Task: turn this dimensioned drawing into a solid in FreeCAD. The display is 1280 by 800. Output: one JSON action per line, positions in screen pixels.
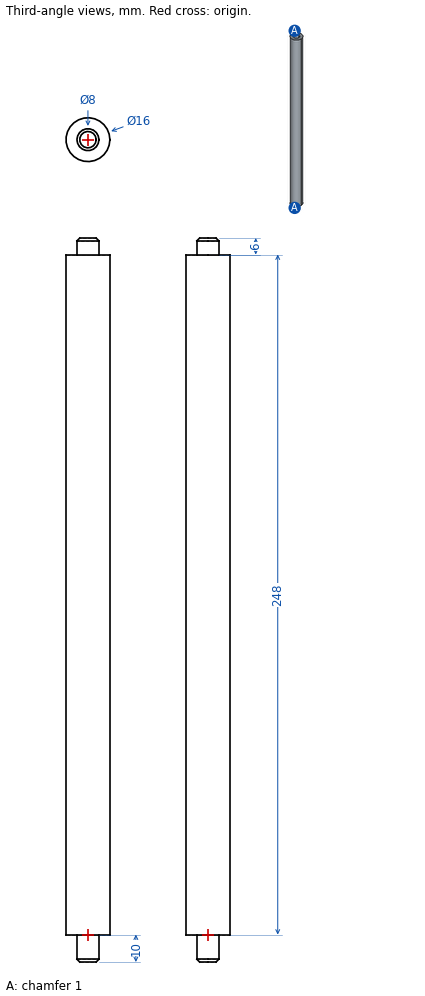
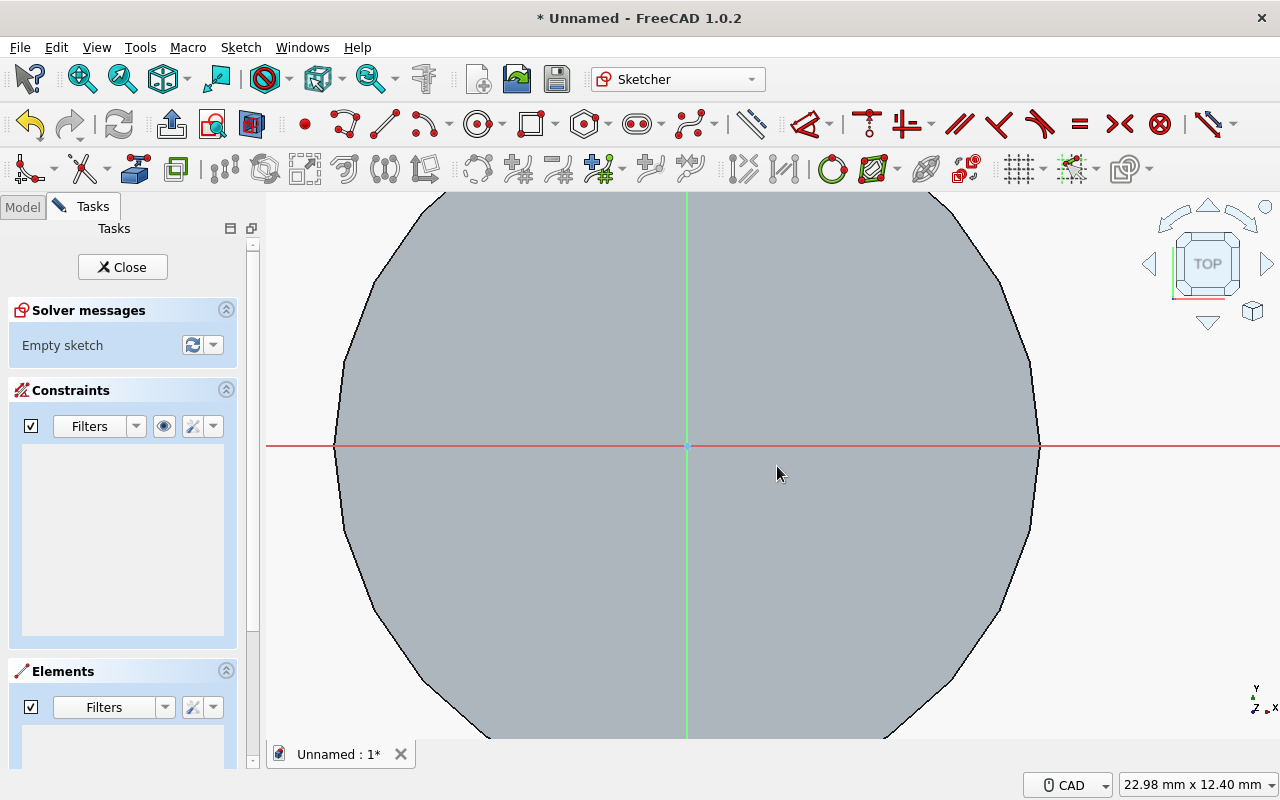
{"action": "key", "text": "g c"}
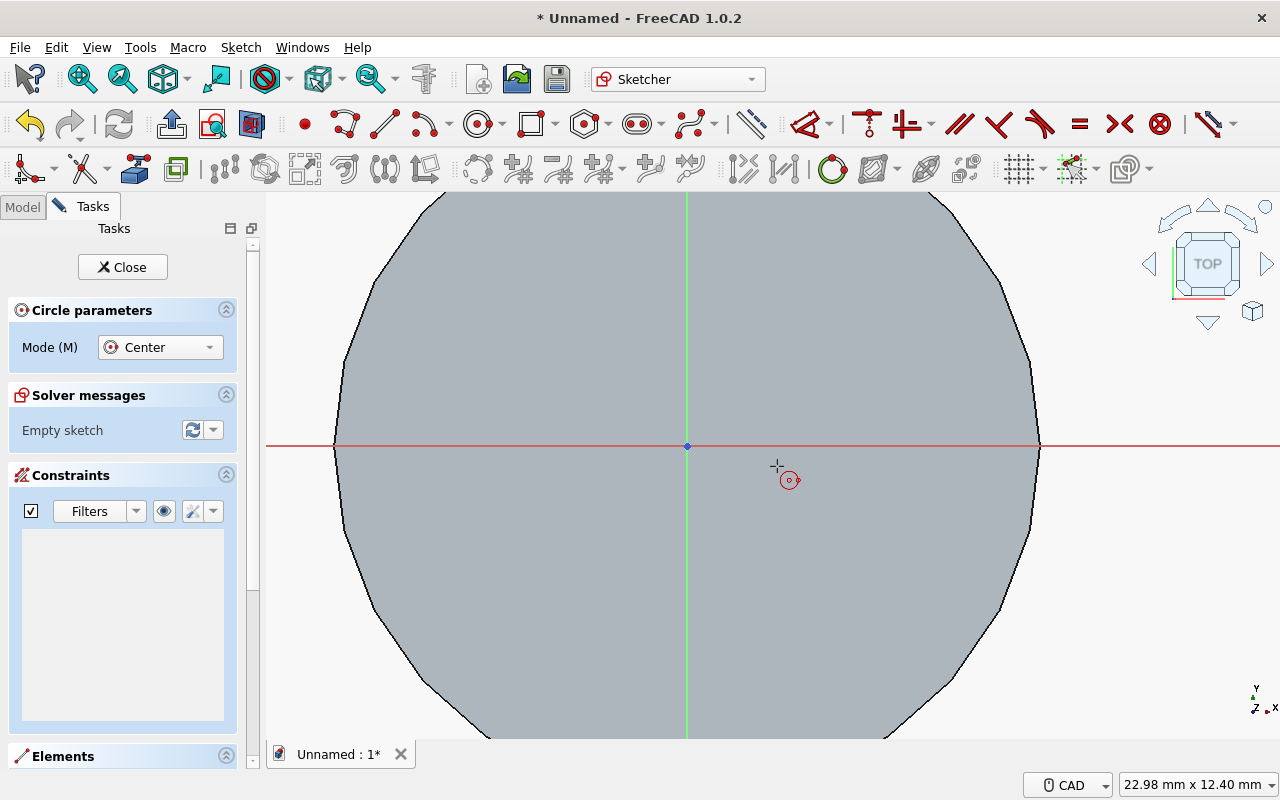
{"action": "left_click", "coordinate": [687, 446]}
{"action": "left_click", "coordinate": [812, 322]}
{"action": "key", "text": "Escape"}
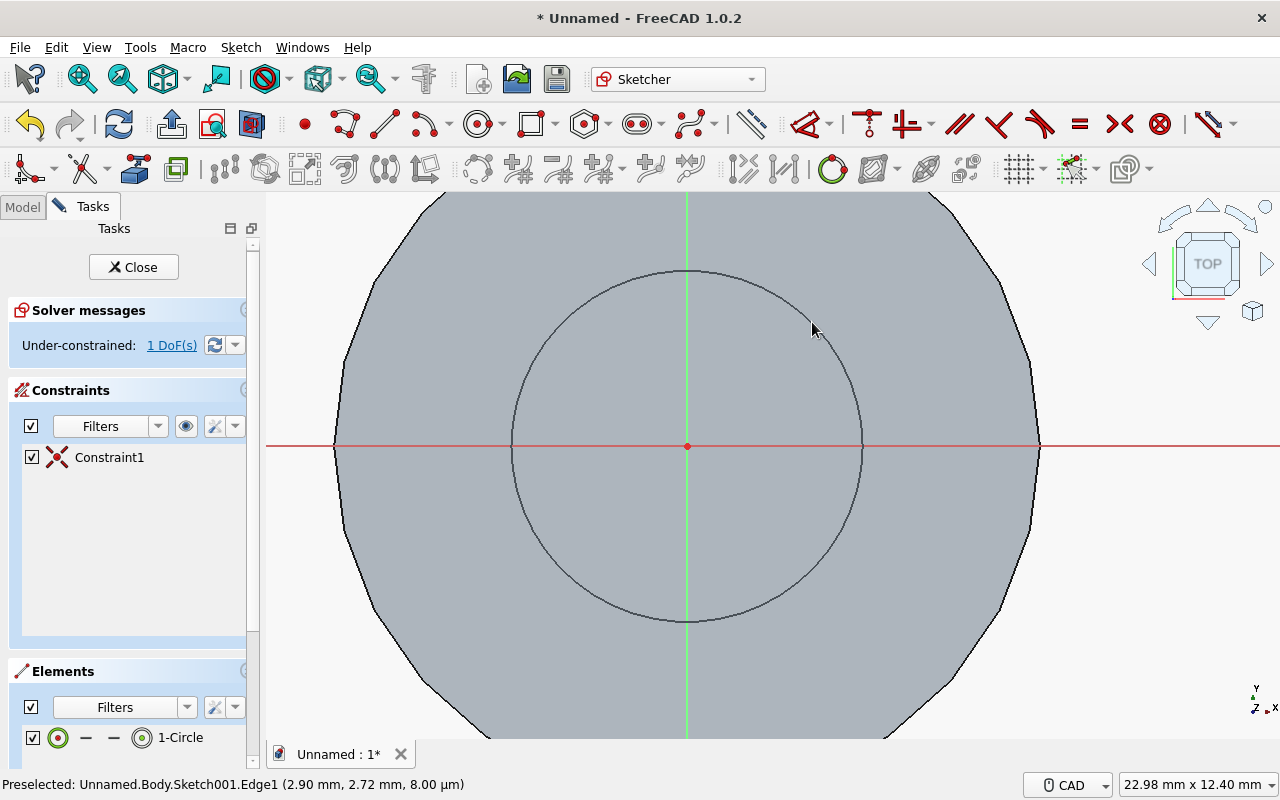
{"action": "left_click", "coordinate": [806, 124]}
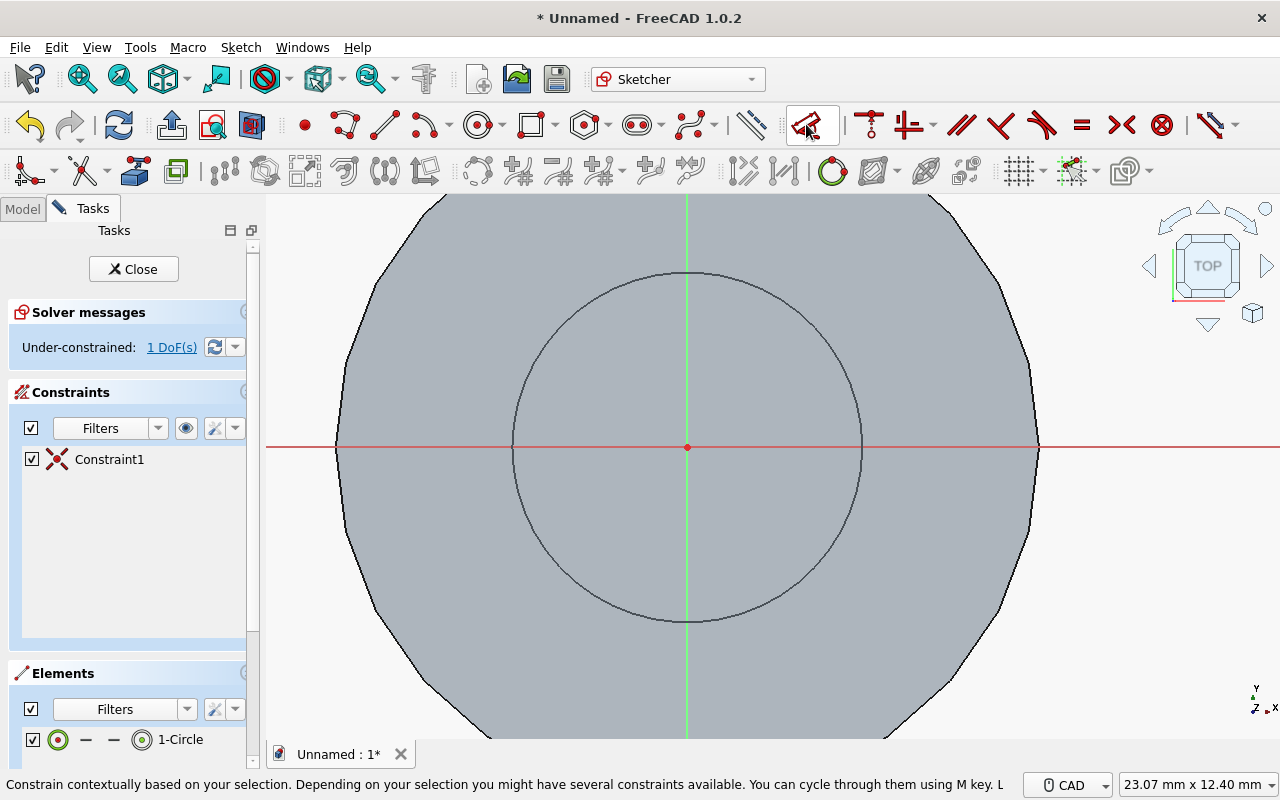
{"action": "left_click", "coordinate": [811, 323]}
{"action": "left_click", "coordinate": [834, 300]}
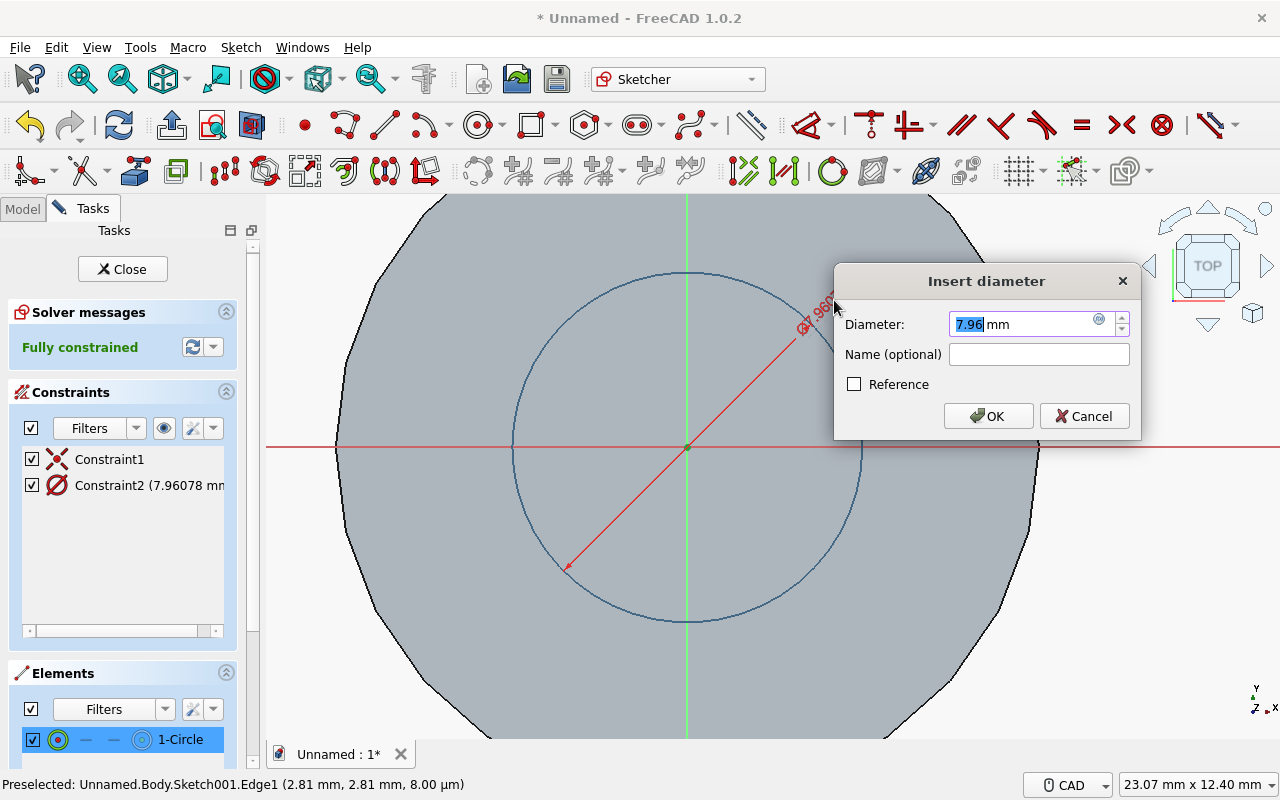
{"action": "type", "text": "8"}
{"action": "key", "text": "Return"}
{"action": "key", "text": "Escape"}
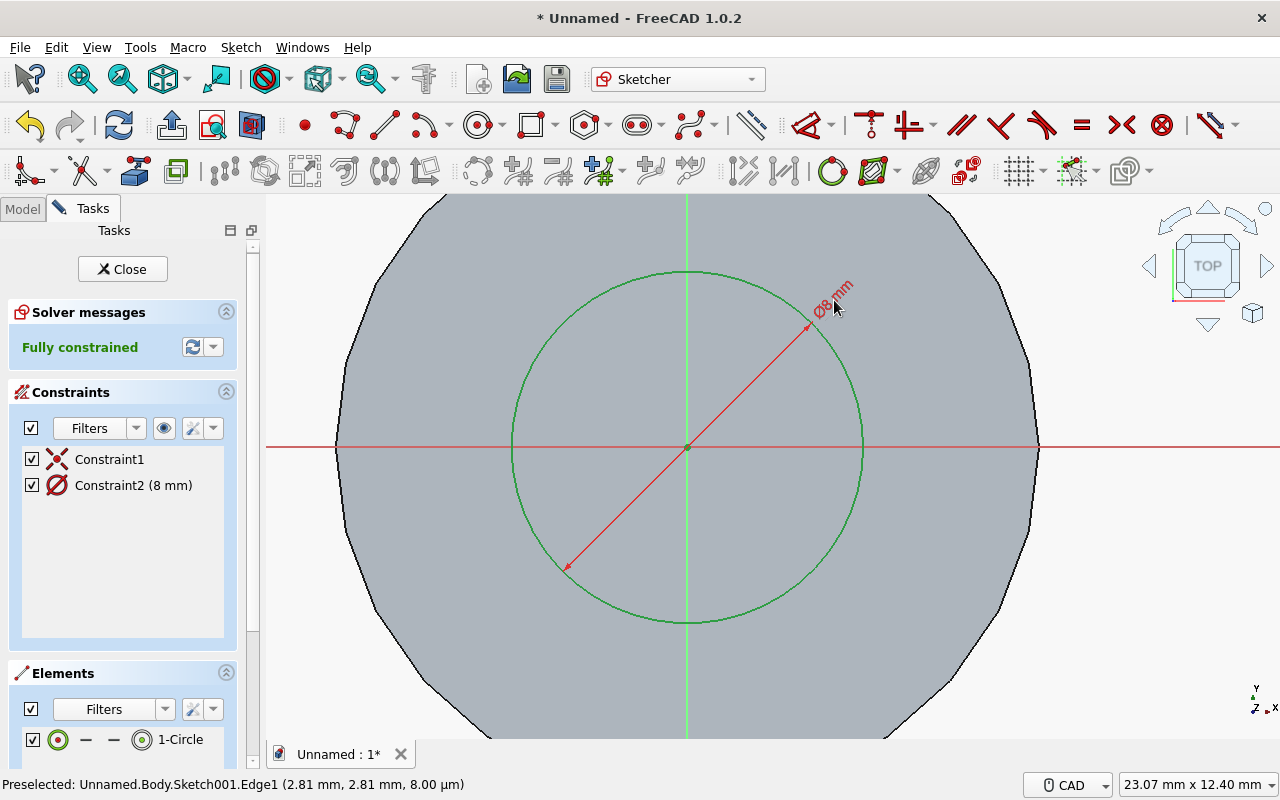
{"action": "left_click", "coordinate": [123, 269]}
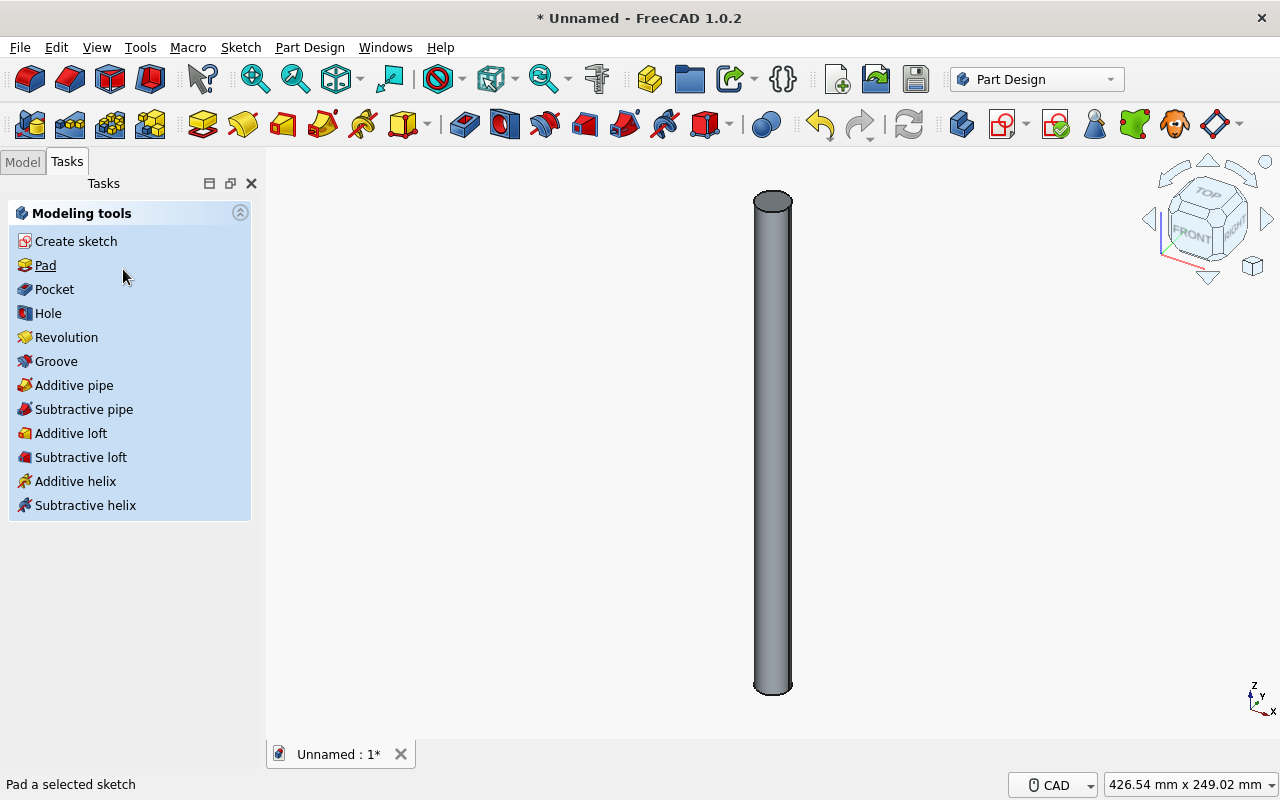
{"action": "left_click", "coordinate": [204, 124]}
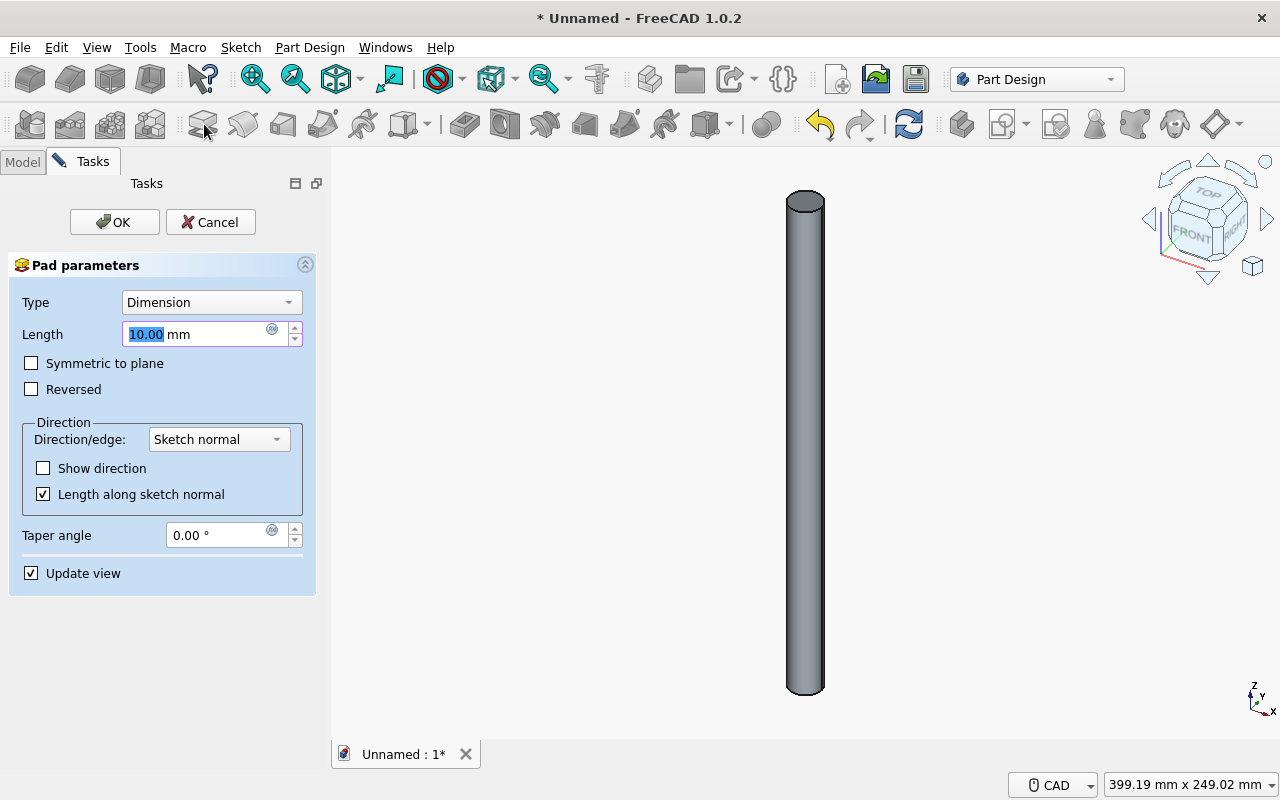
{"action": "type", "text": "10"}
{"action": "key", "text": "Tab"}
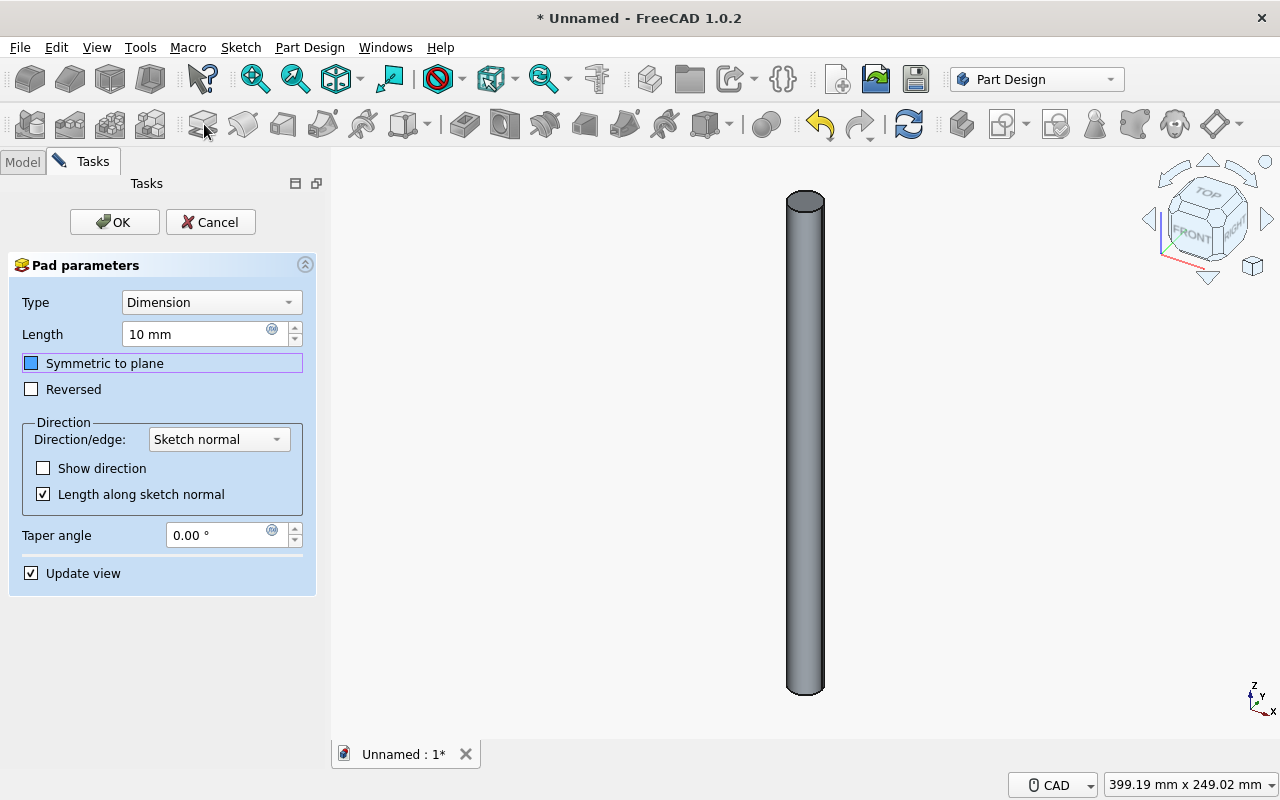
{"action": "left_click", "coordinate": [30, 389]}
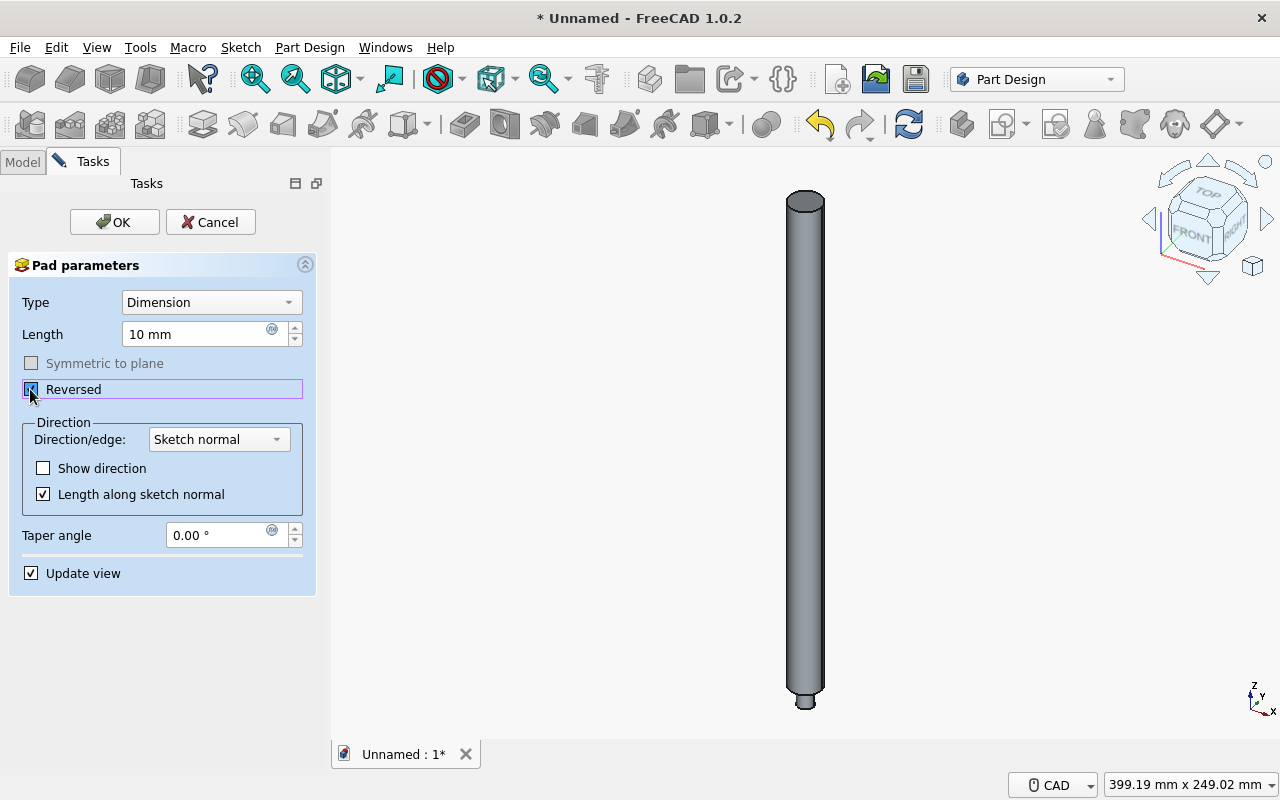
{"action": "left_click", "coordinate": [115, 222]}